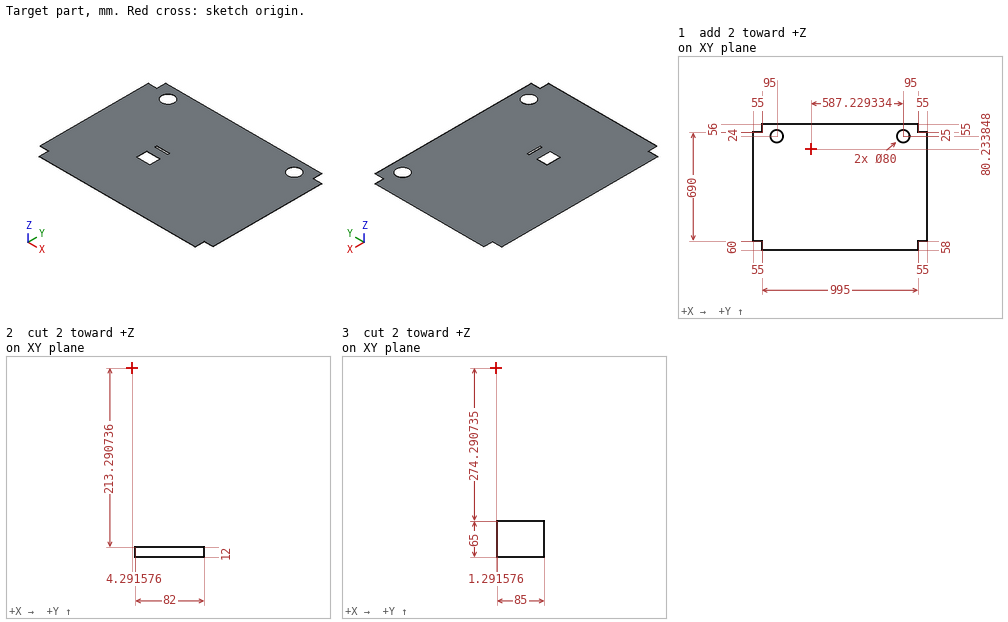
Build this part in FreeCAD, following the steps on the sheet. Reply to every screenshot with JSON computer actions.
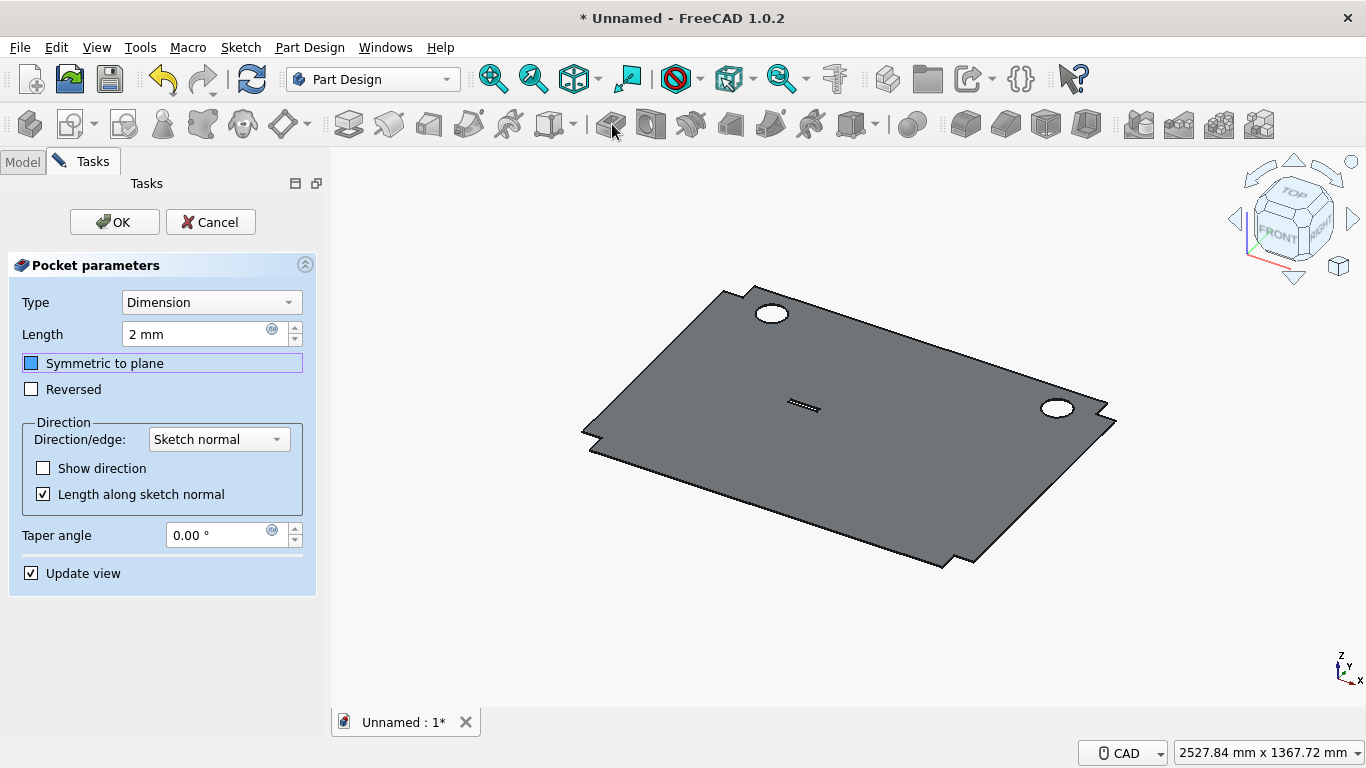
{"action": "left_click", "coordinate": [30, 389]}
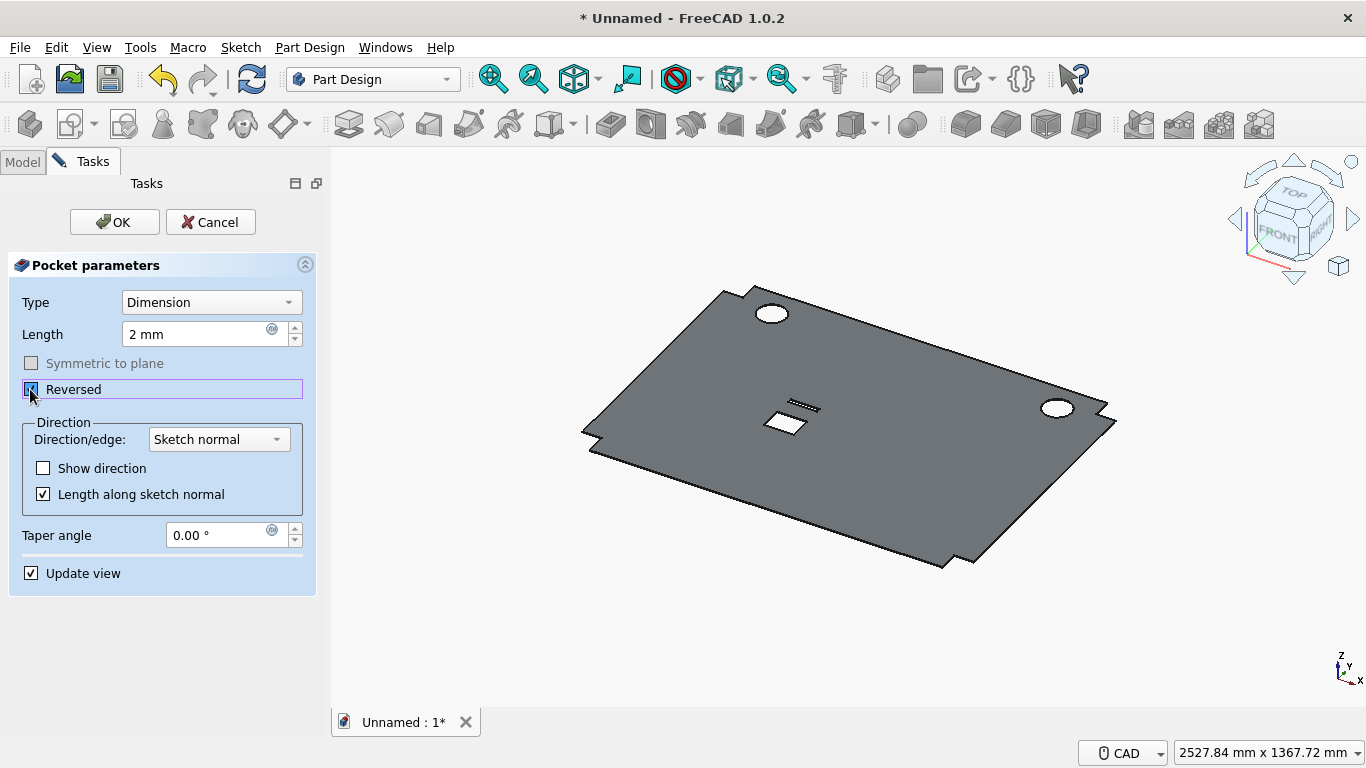
{"action": "left_click", "coordinate": [115, 222]}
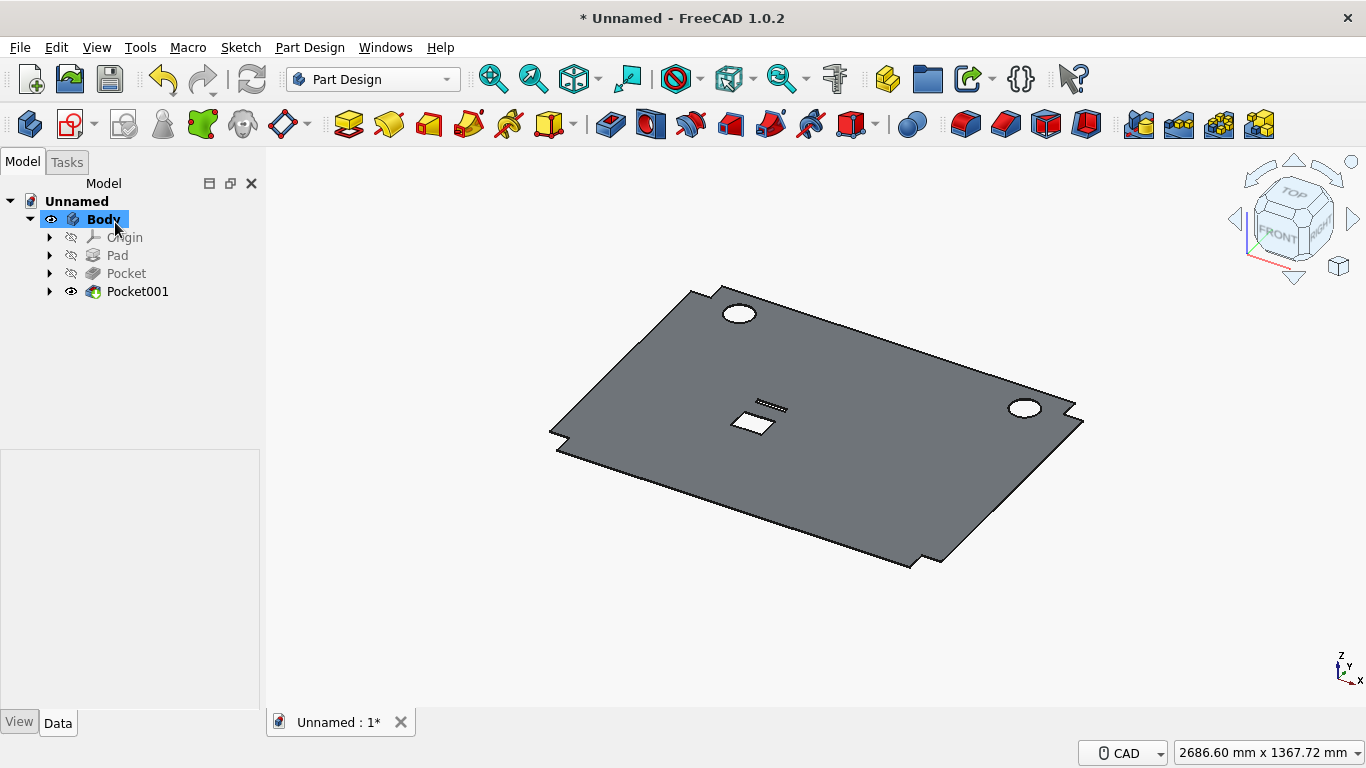
{"action": "key", "text": "0"}